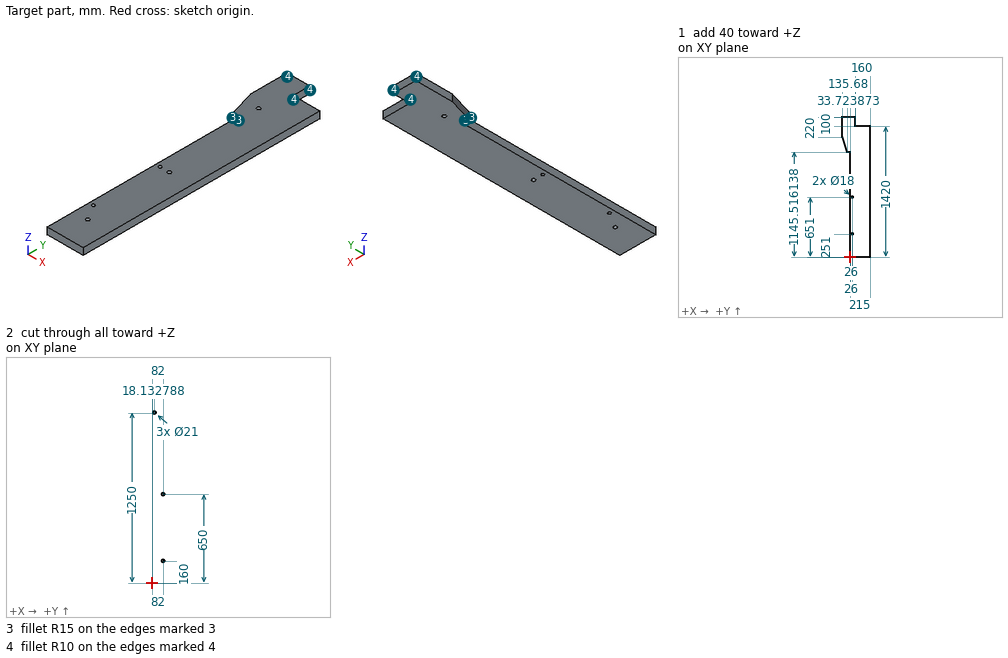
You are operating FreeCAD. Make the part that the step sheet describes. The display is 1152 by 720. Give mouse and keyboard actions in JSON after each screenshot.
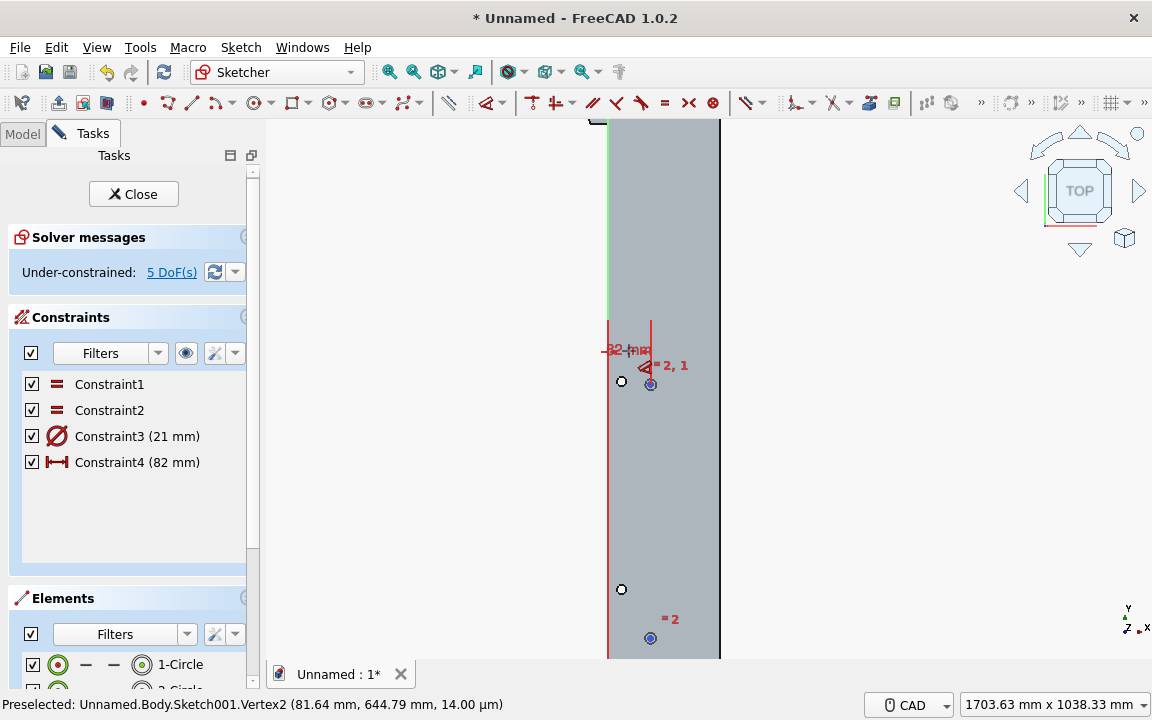
{"action": "scroll", "coordinate": [651, 385], "scroll_direction": "down", "scroll_amount": 3}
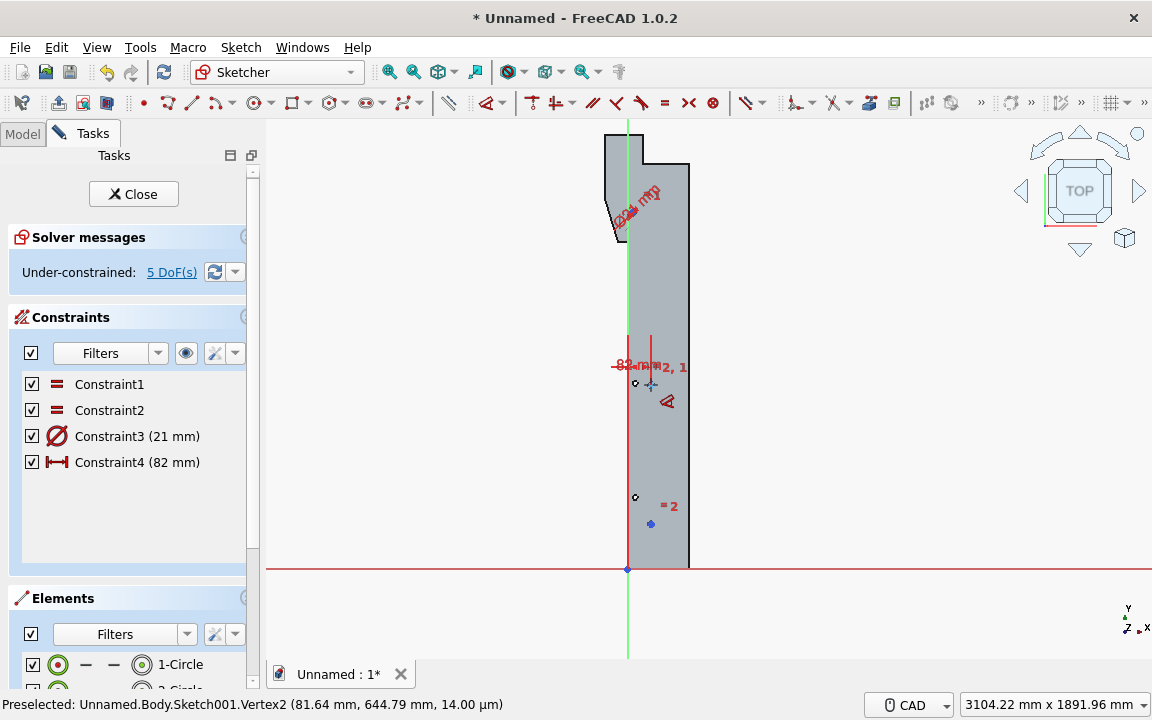
{"action": "scroll", "coordinate": [651, 524], "scroll_direction": "up", "scroll_amount": 3}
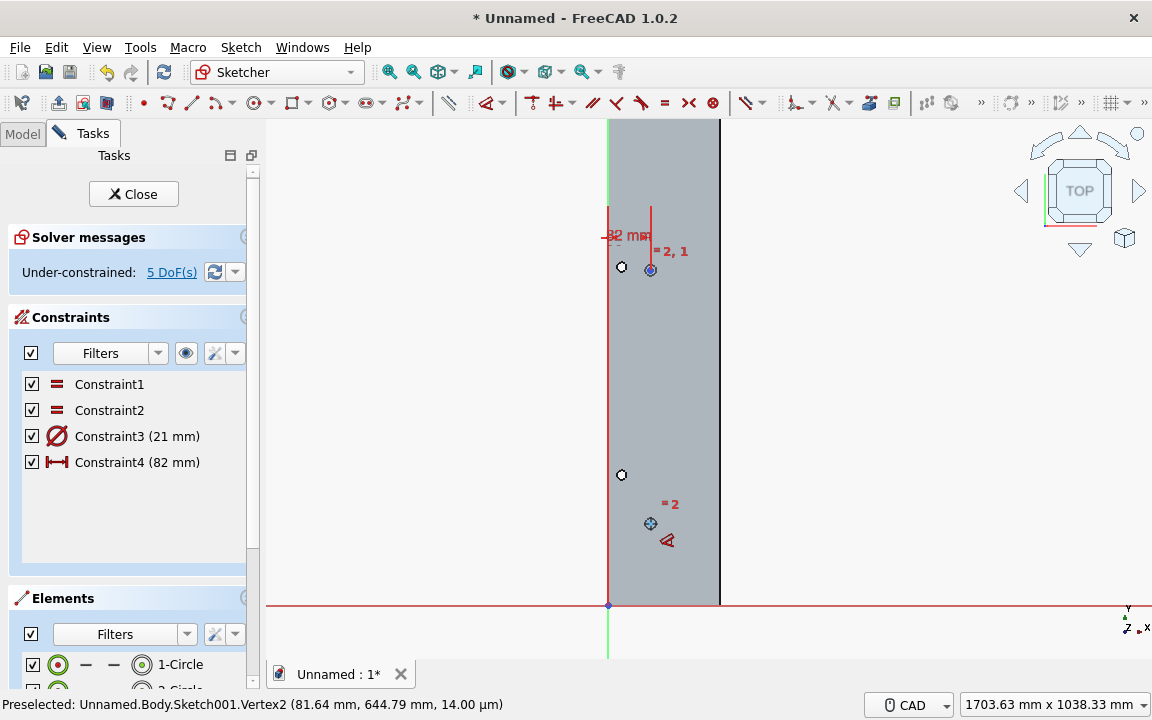
{"action": "left_click", "coordinate": [651, 524]}
{"action": "left_click", "coordinate": [629, 490]}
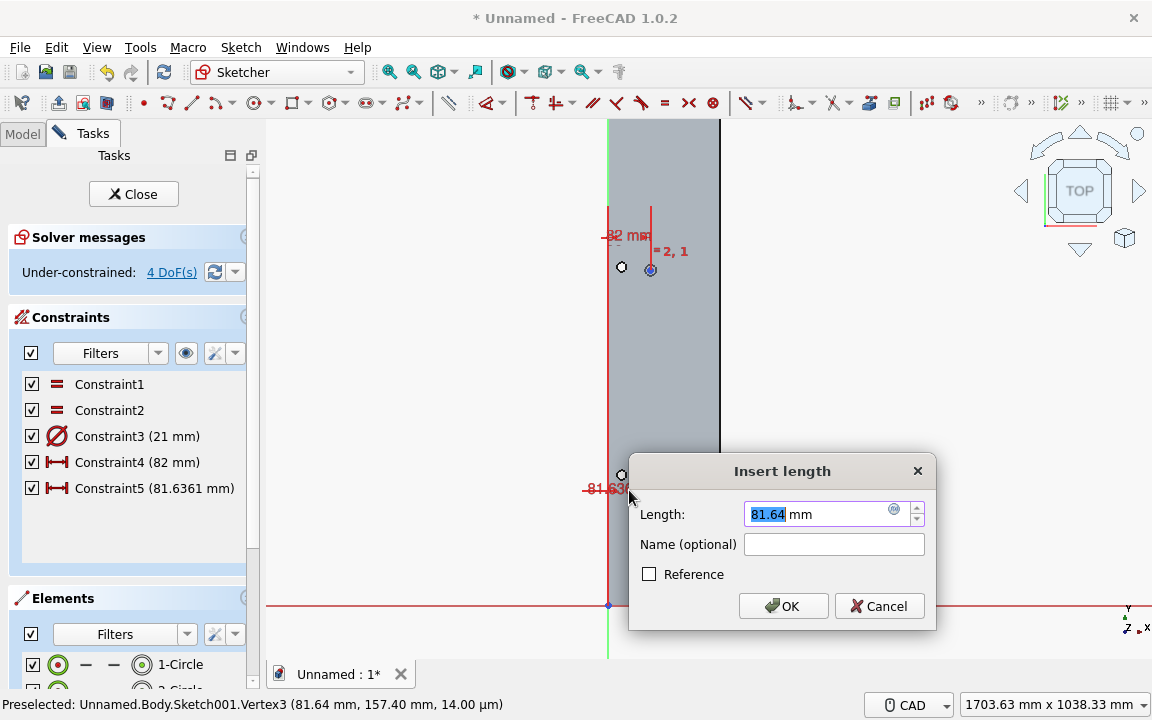
{"action": "type", "text": "82"}
{"action": "key", "text": "Return"}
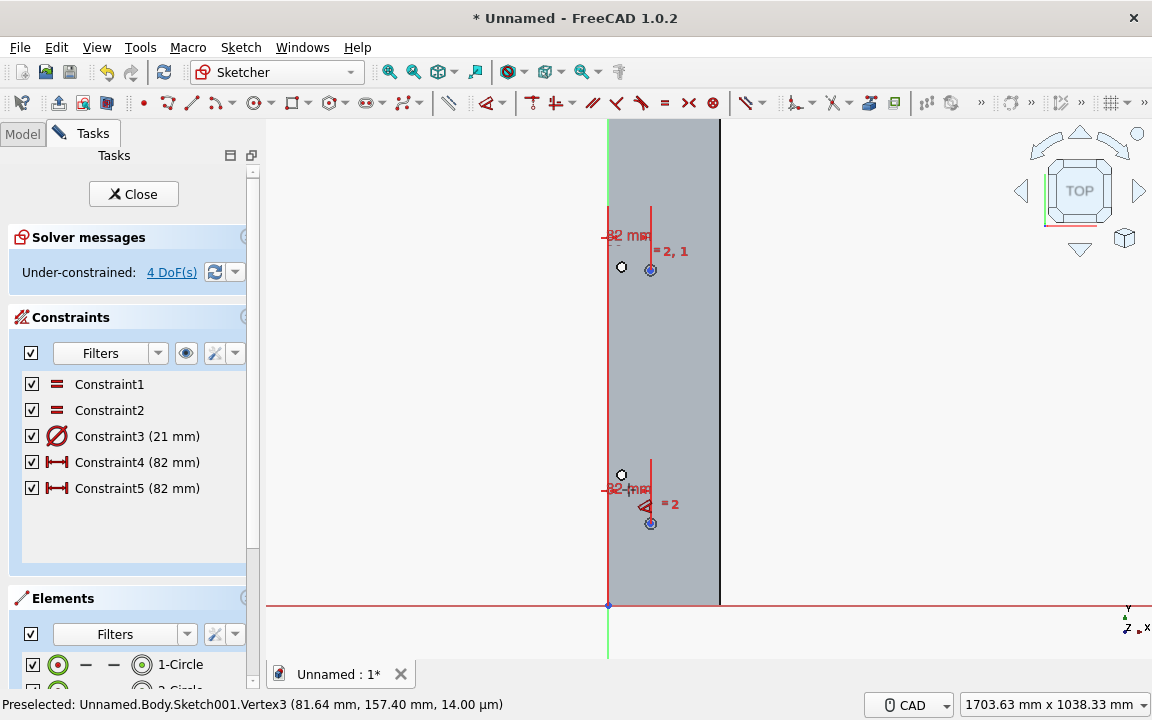
{"action": "left_click", "coordinate": [651, 270]}
{"action": "left_click", "coordinate": [574, 438]}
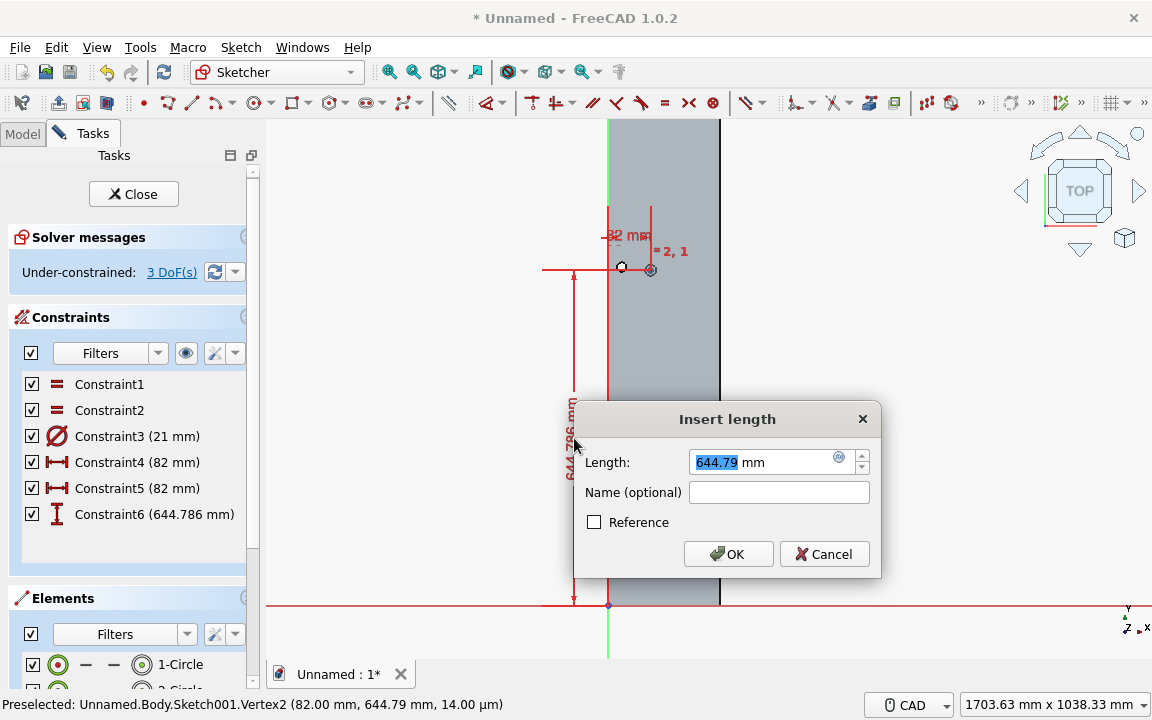
{"action": "type", "text": "650"}
{"action": "key", "text": "Return"}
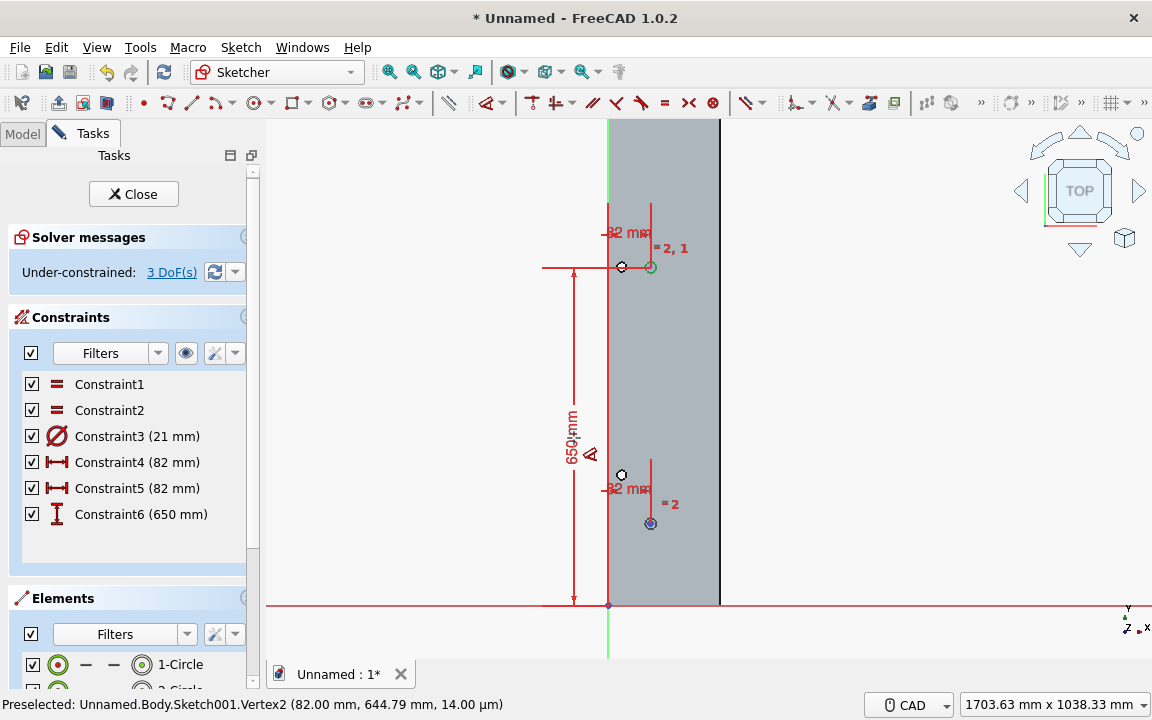
{"action": "left_click", "coordinate": [651, 524]}
{"action": "left_click", "coordinate": [574, 565]}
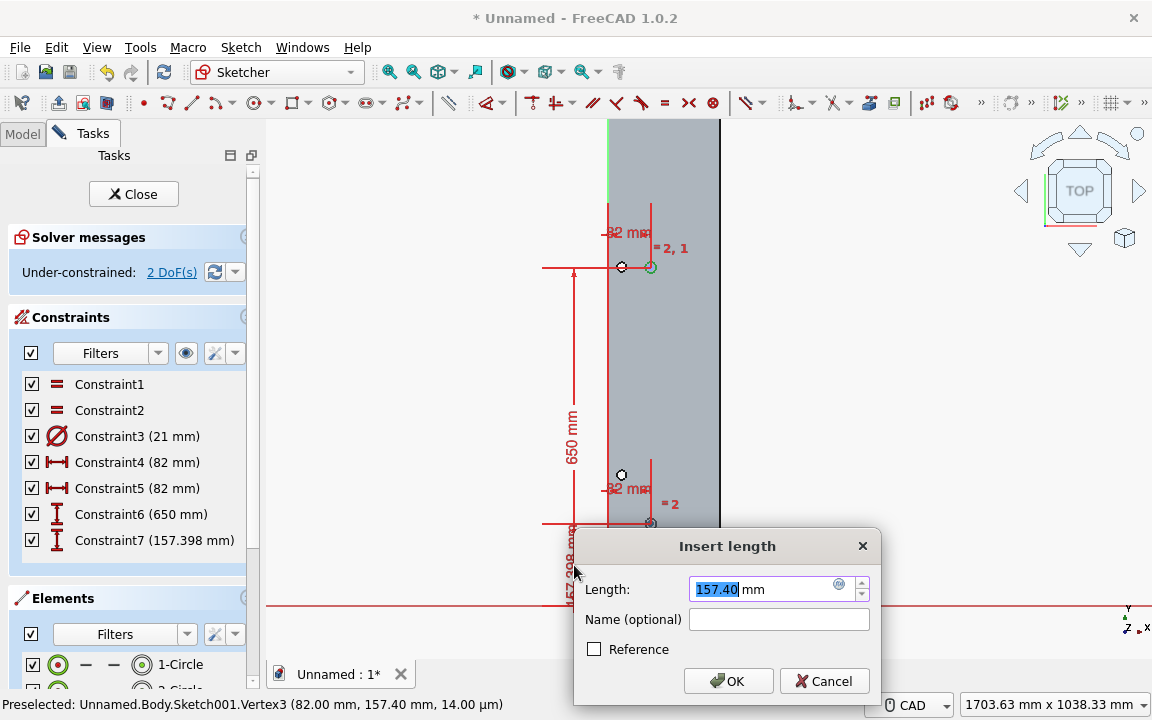
{"action": "type", "text": "160"}
{"action": "key", "text": "Return"}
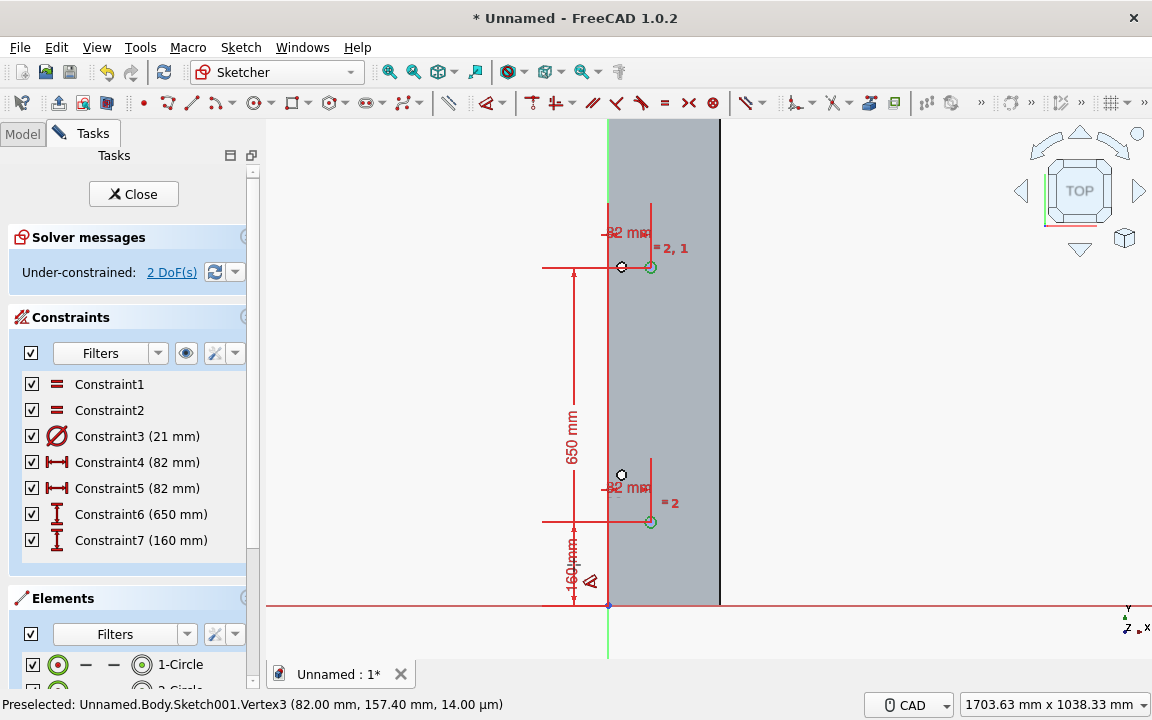
{"action": "scroll", "coordinate": [651, 524], "scroll_direction": "down", "scroll_amount": 3}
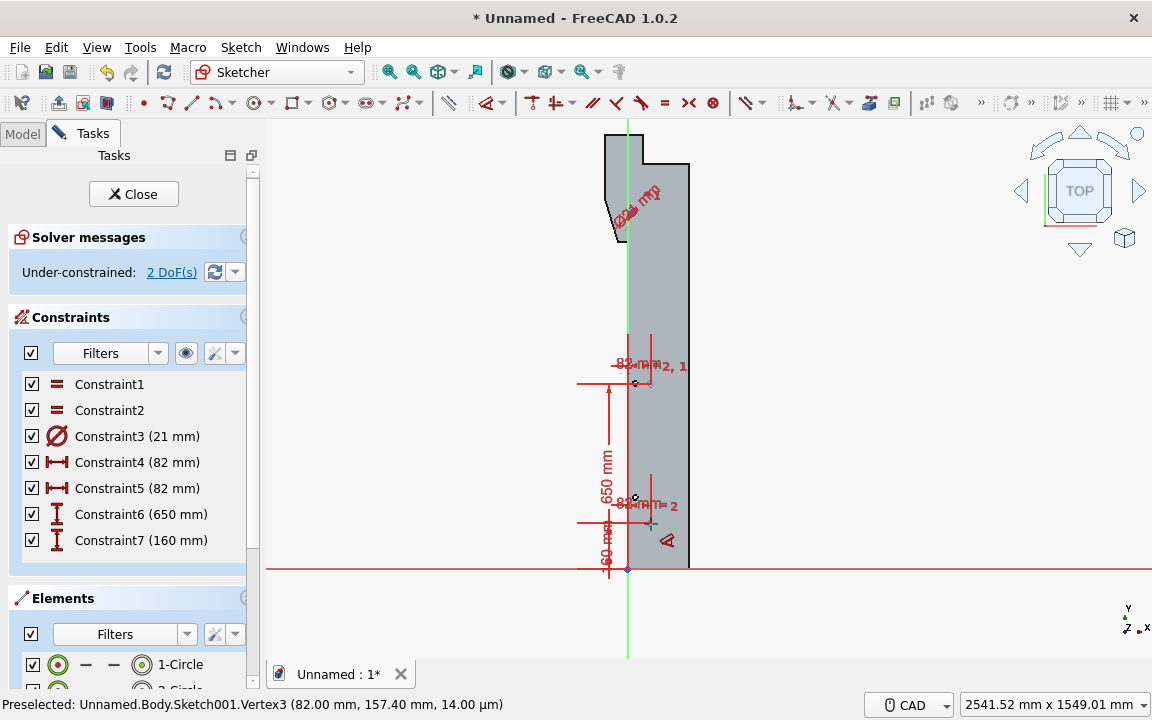
{"action": "left_click", "coordinate": [633, 213]}
{"action": "left_click", "coordinate": [594, 391]}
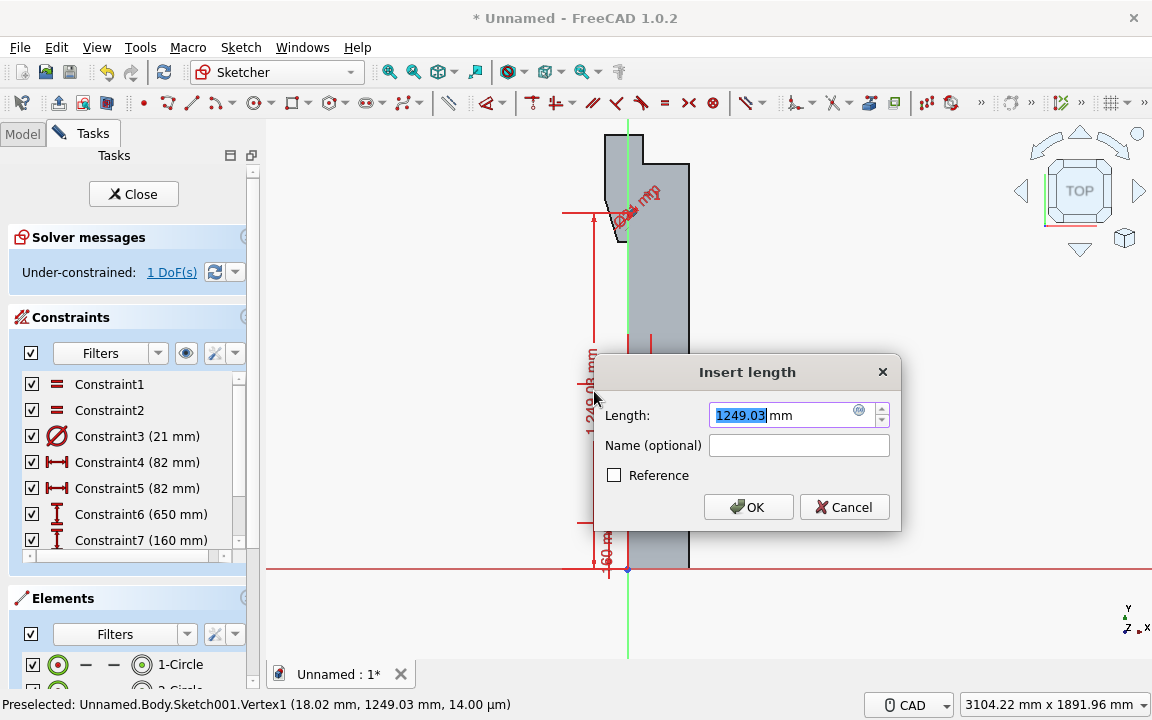
{"action": "type", "text": "1250"}
{"action": "key", "text": "Return"}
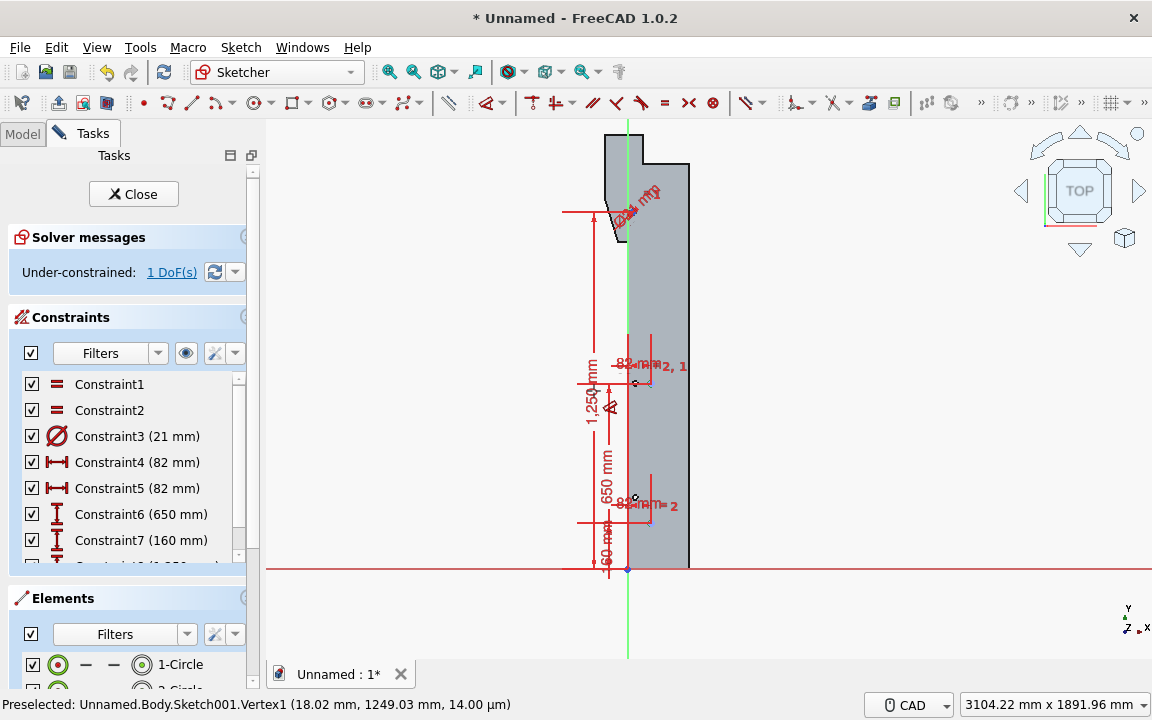
{"action": "scroll", "coordinate": [633, 212], "scroll_direction": "up", "scroll_amount": 11}